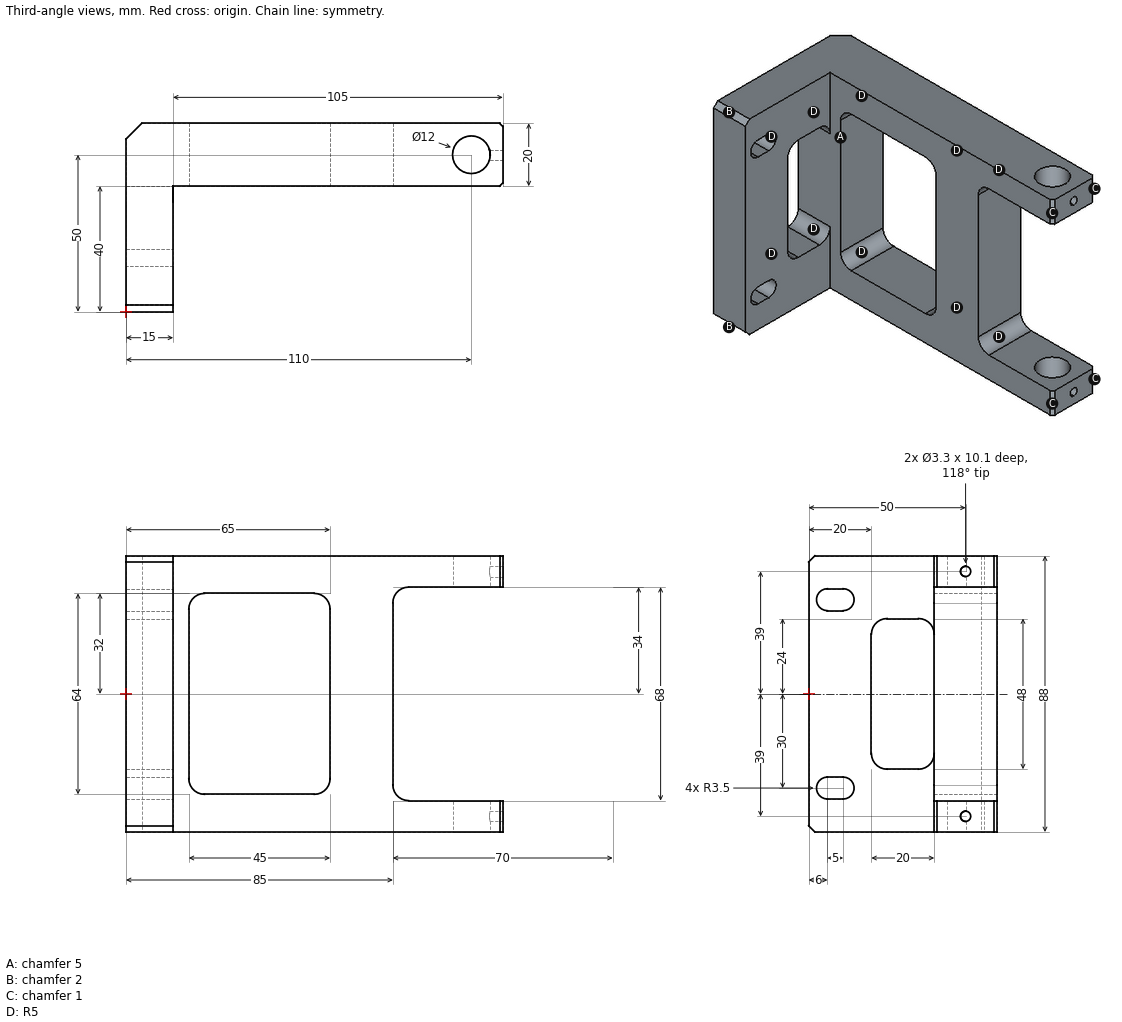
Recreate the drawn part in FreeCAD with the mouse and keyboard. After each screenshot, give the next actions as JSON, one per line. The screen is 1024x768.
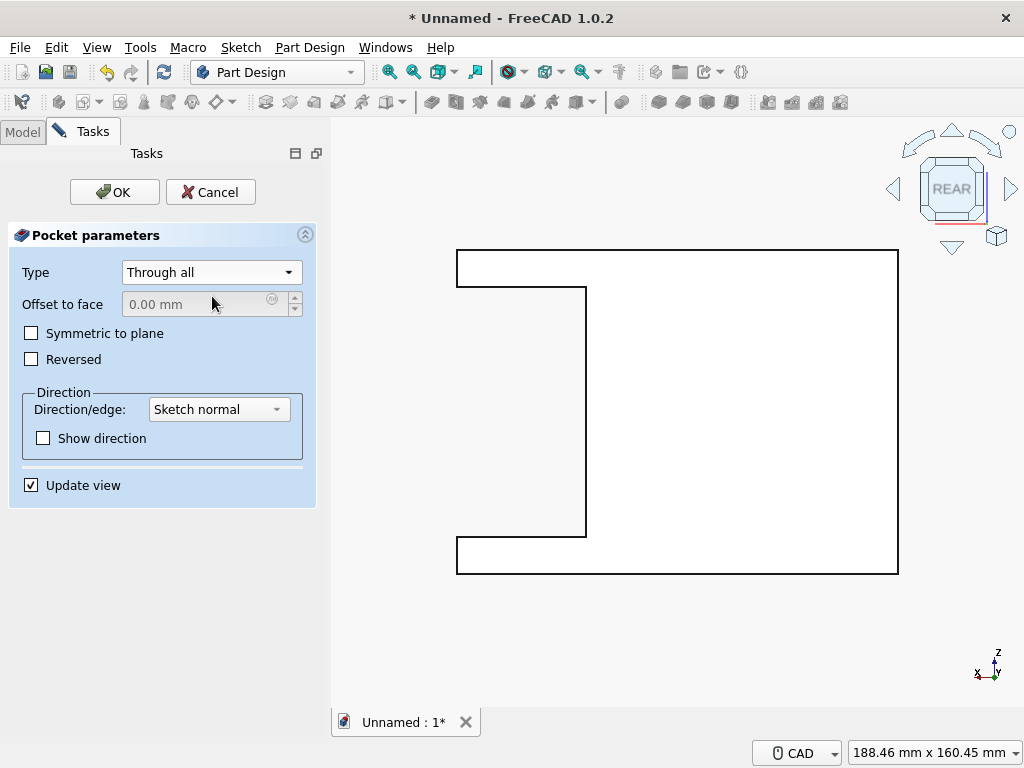
{"action": "left_click", "coordinate": [115, 192]}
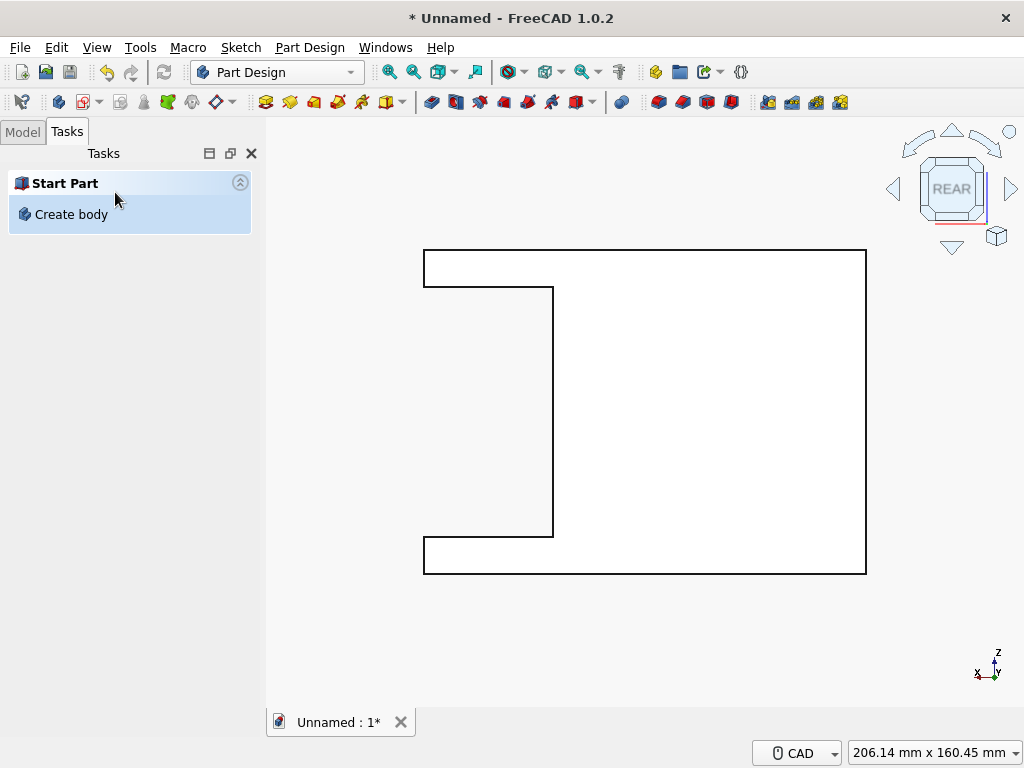
{"action": "key", "text": "6"}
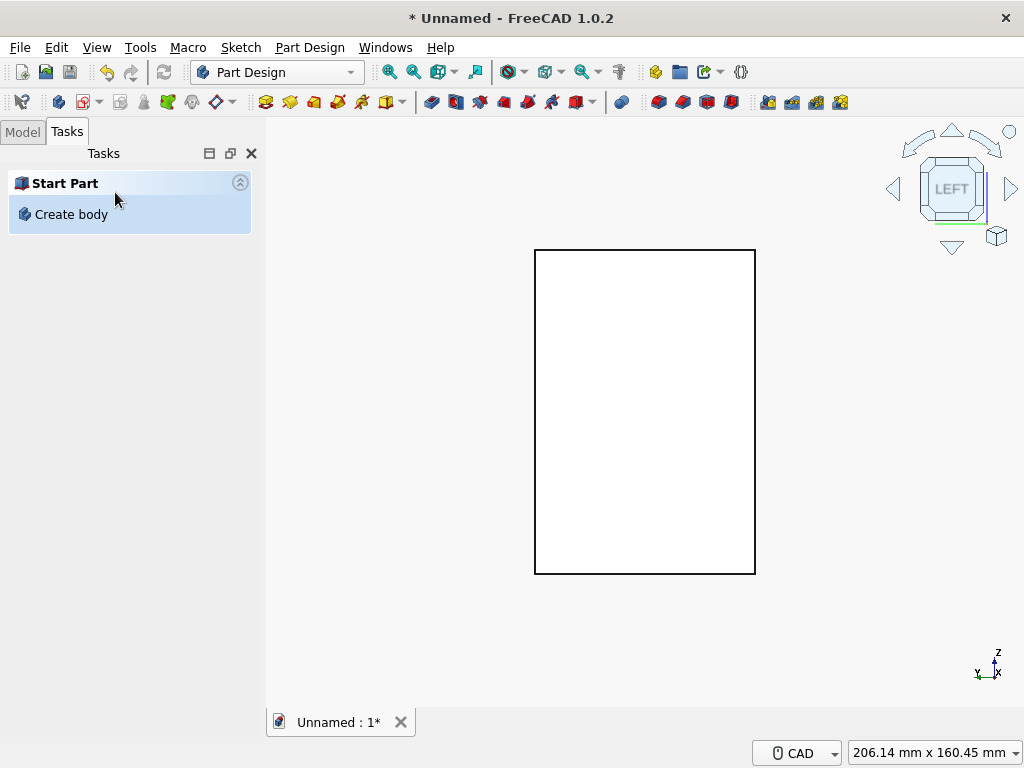
{"action": "left_click", "coordinate": [645, 365]}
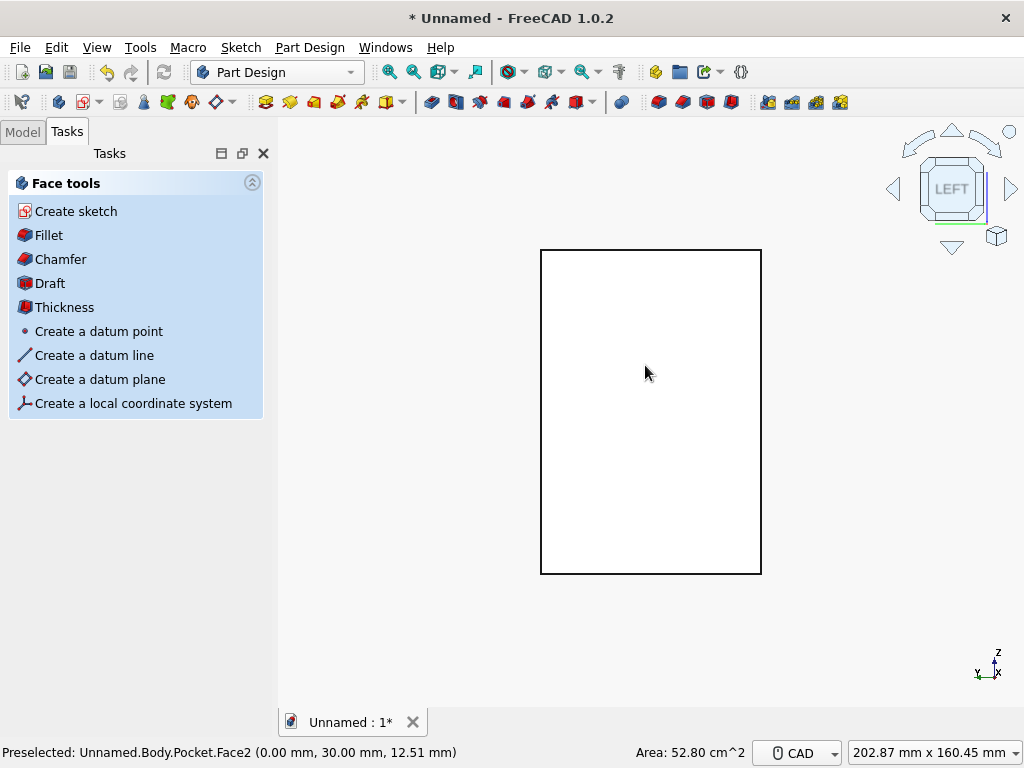
{"action": "left_click", "coordinate": [84, 102]}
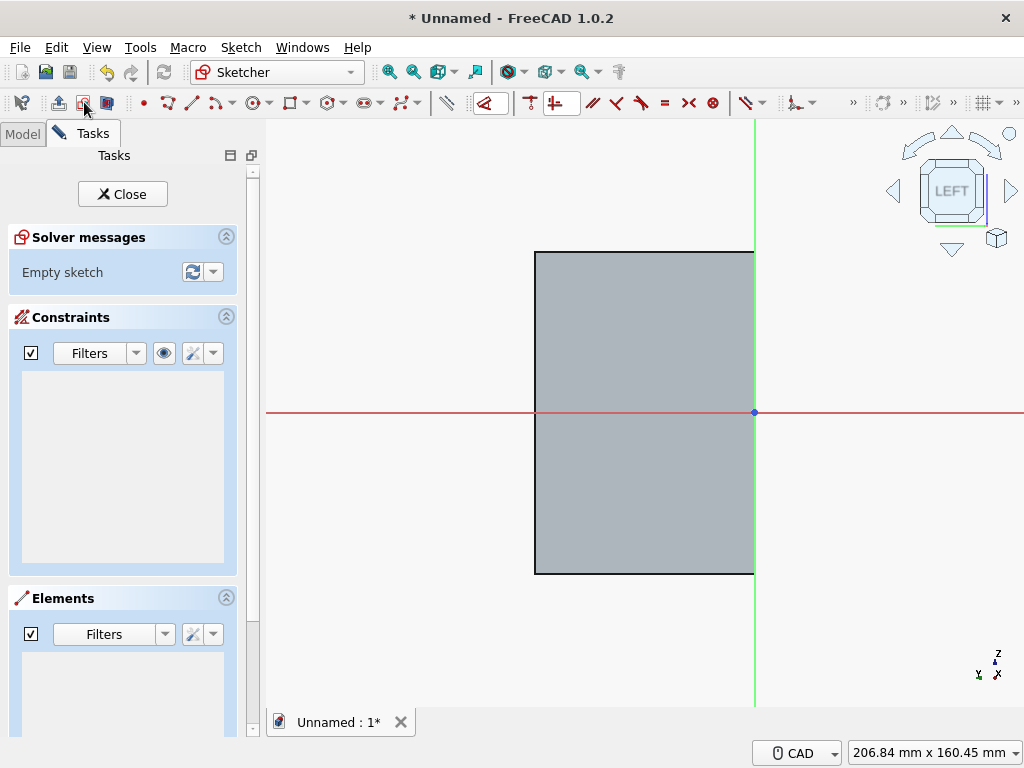
{"action": "scroll", "coordinate": [859, 413], "scroll_direction": "up", "scroll_amount": 2}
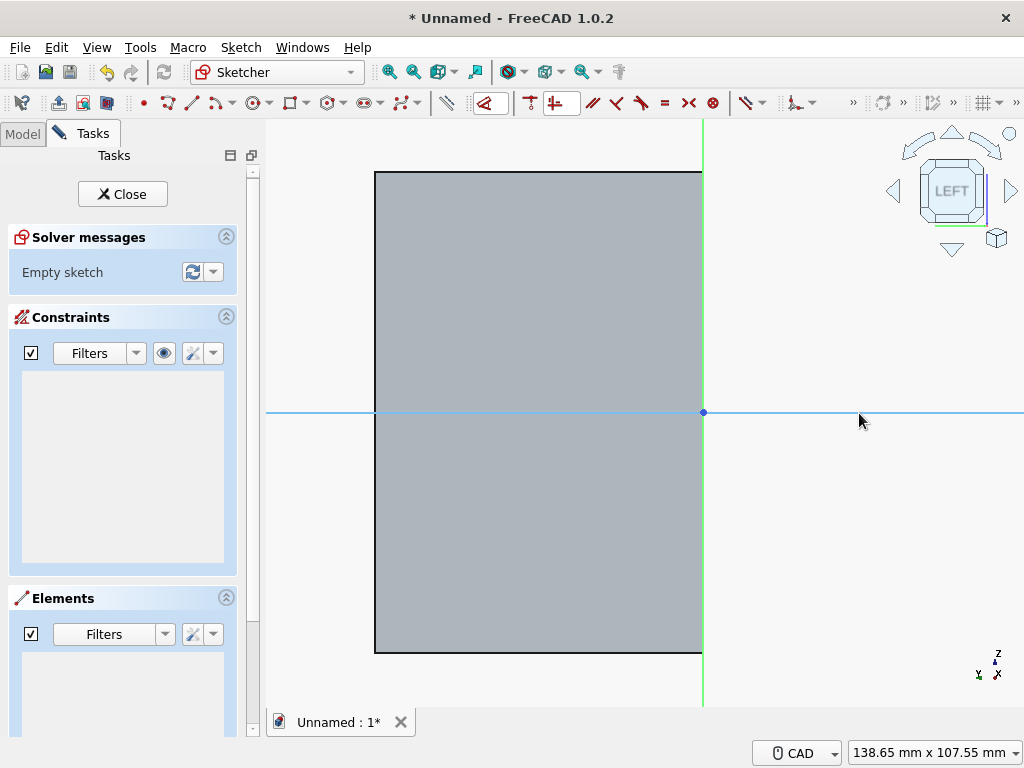
{"action": "key", "text": "g s"}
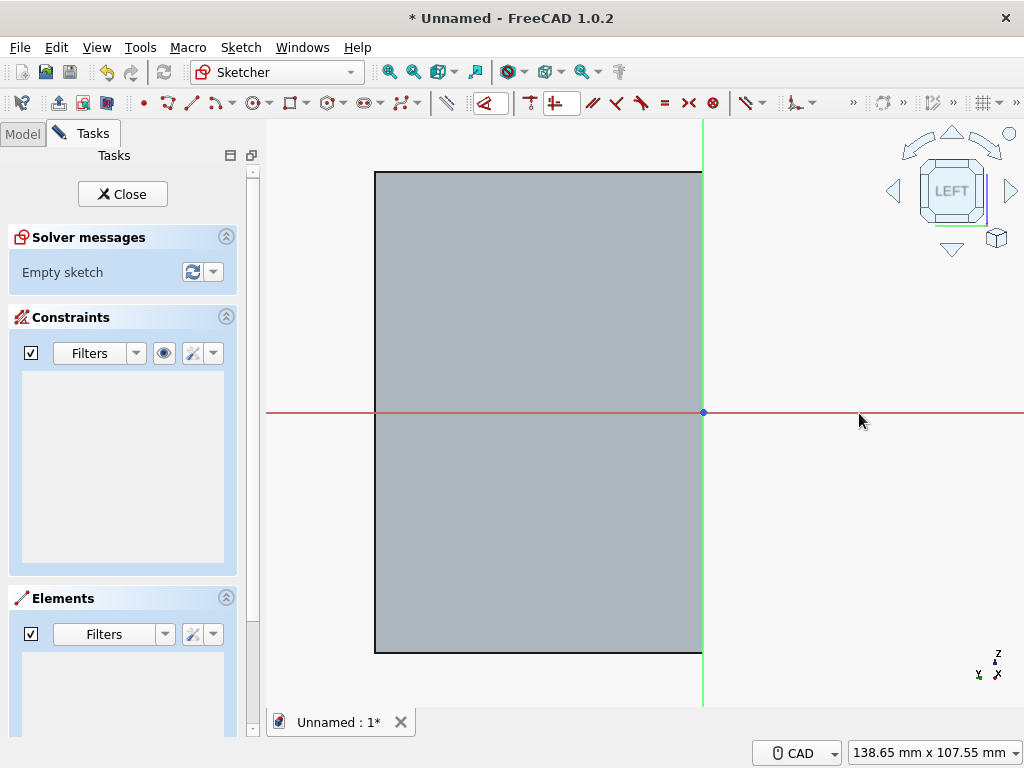
{"action": "left_click", "coordinate": [643, 577]}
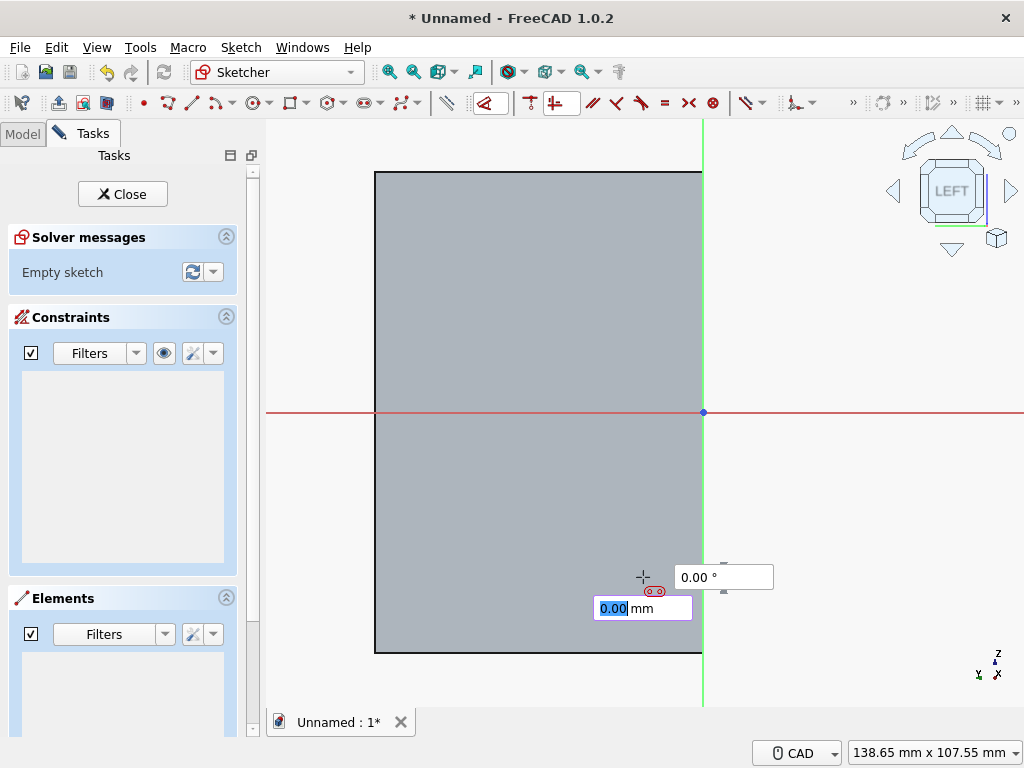
{"action": "left_click", "coordinate": [671, 577]}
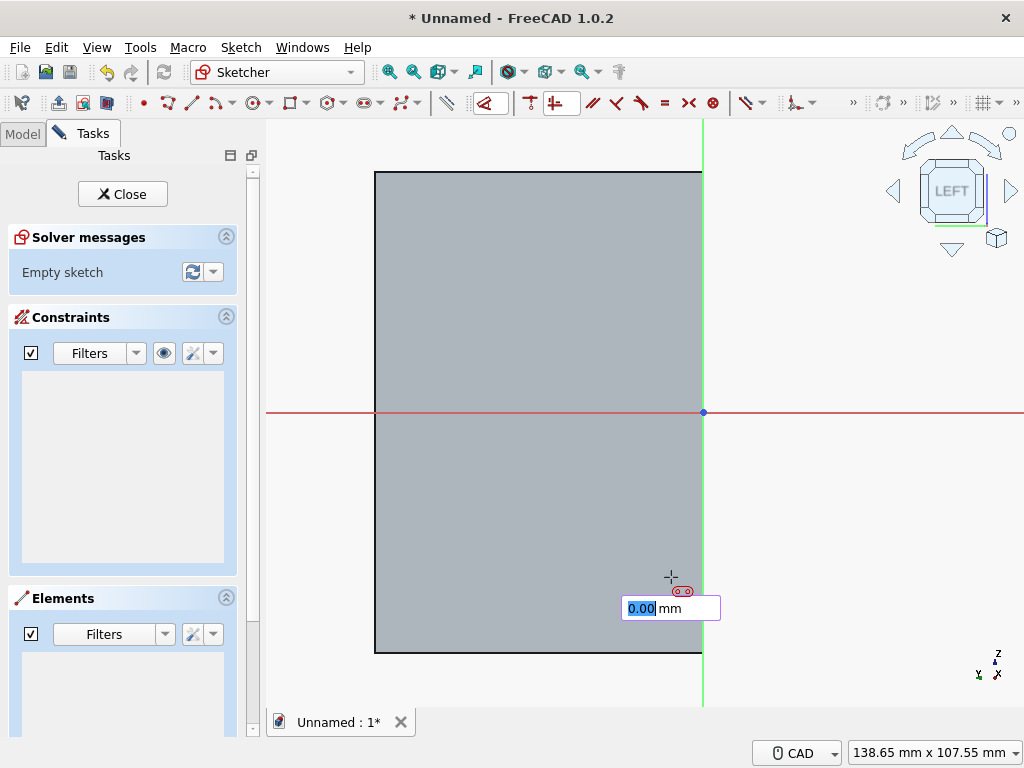
{"action": "left_click", "coordinate": [657, 596]}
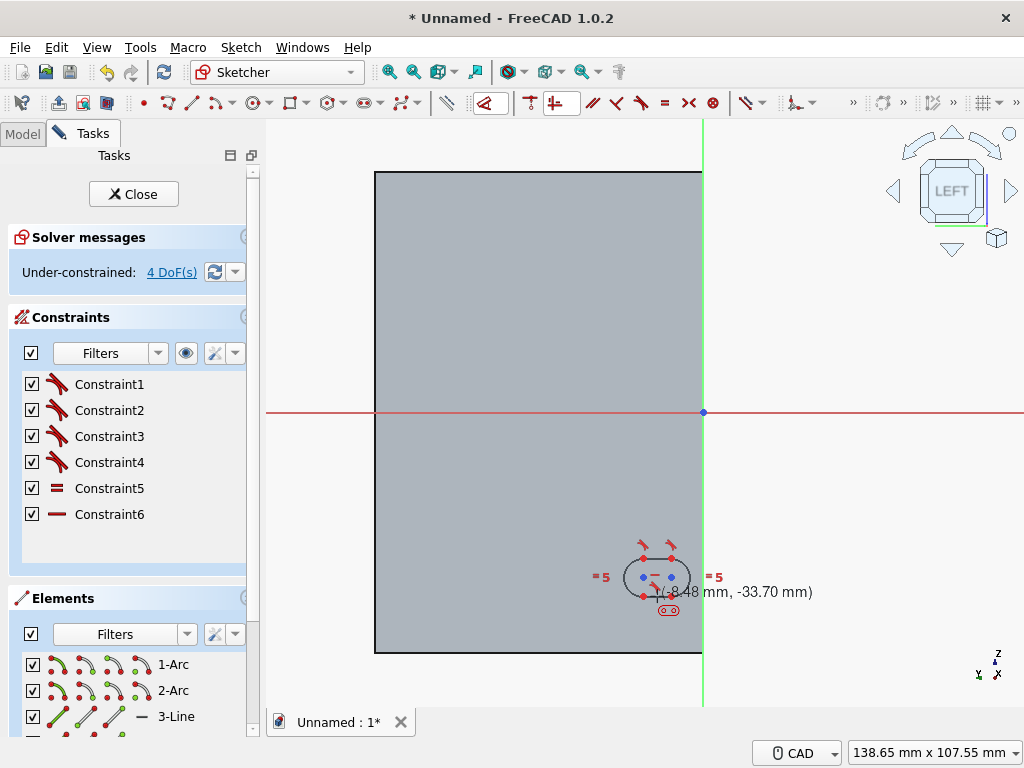
{"action": "left_click", "coordinate": [643, 249]}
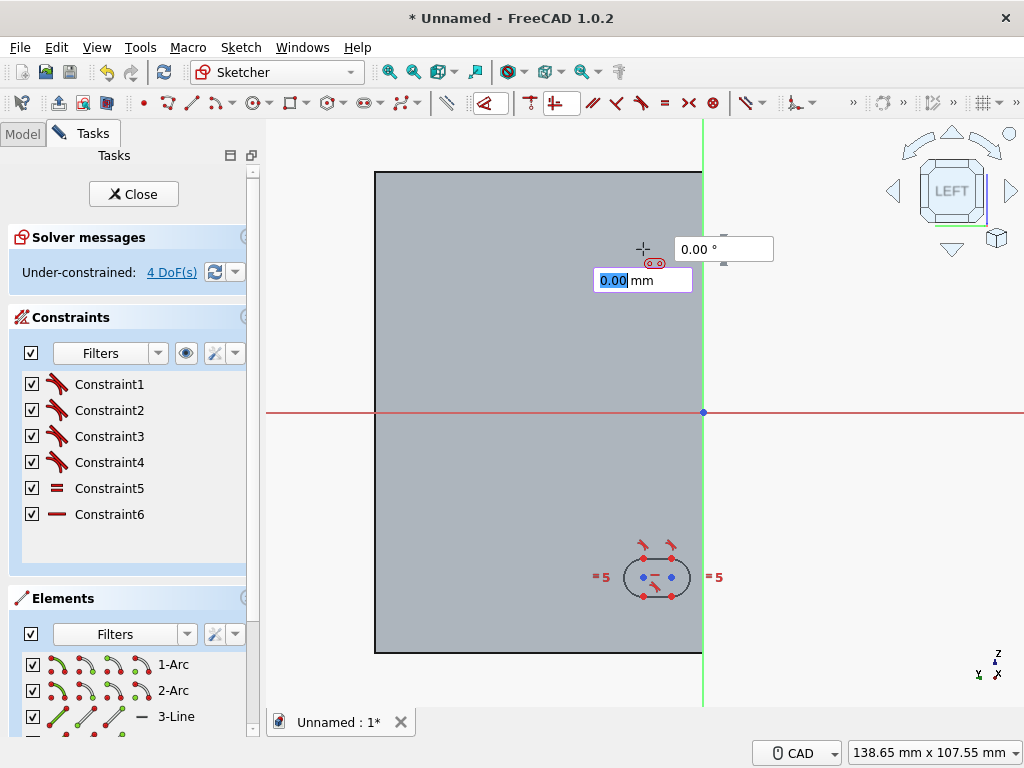
{"action": "left_click", "coordinate": [671, 249]}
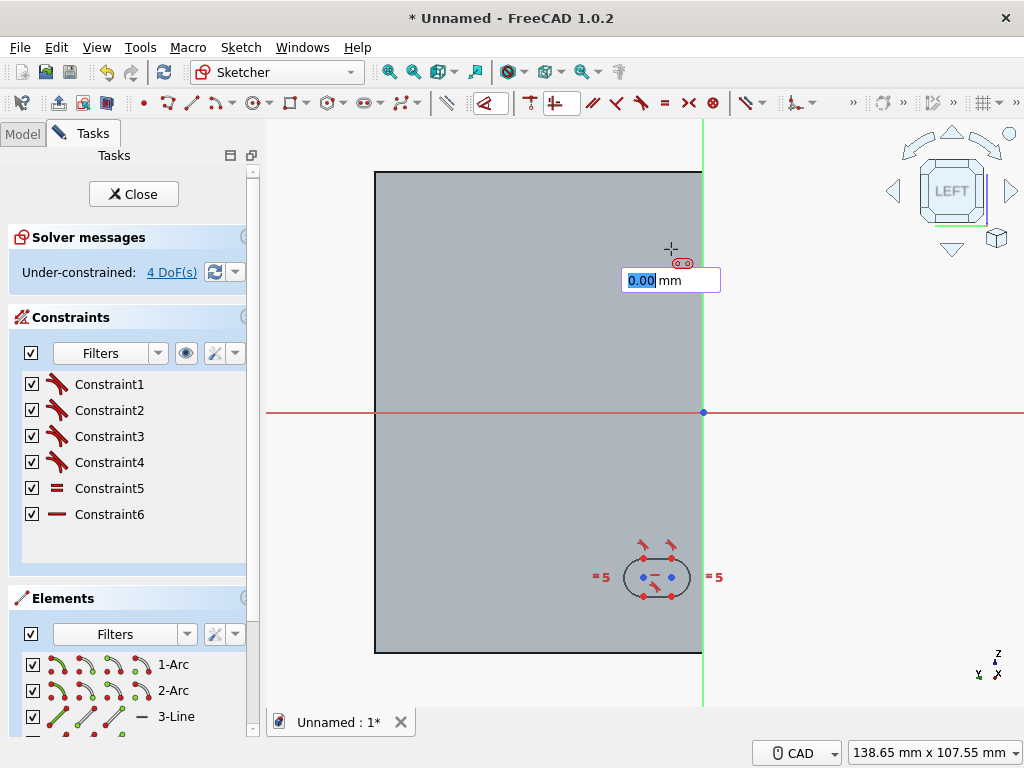
{"action": "left_click", "coordinate": [657, 230]}
{"action": "key", "text": "Escape"}